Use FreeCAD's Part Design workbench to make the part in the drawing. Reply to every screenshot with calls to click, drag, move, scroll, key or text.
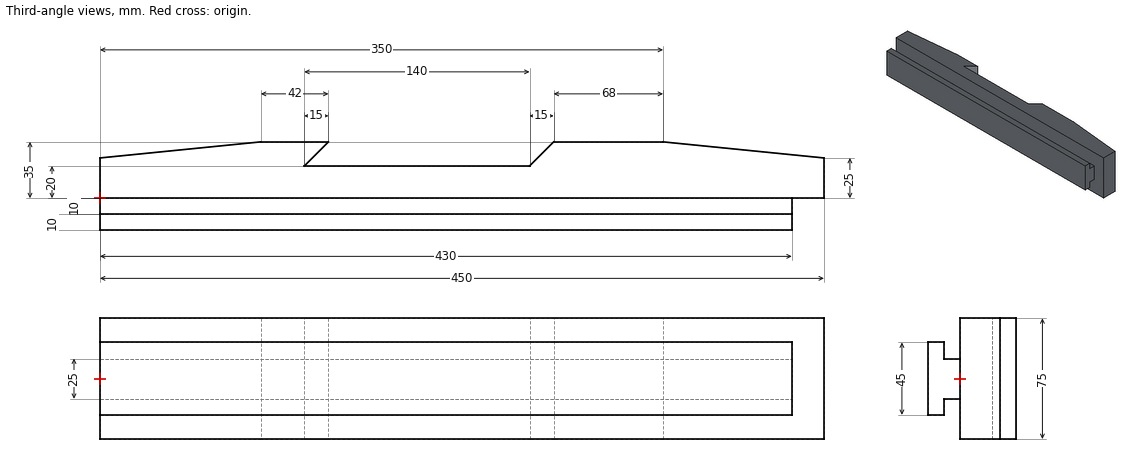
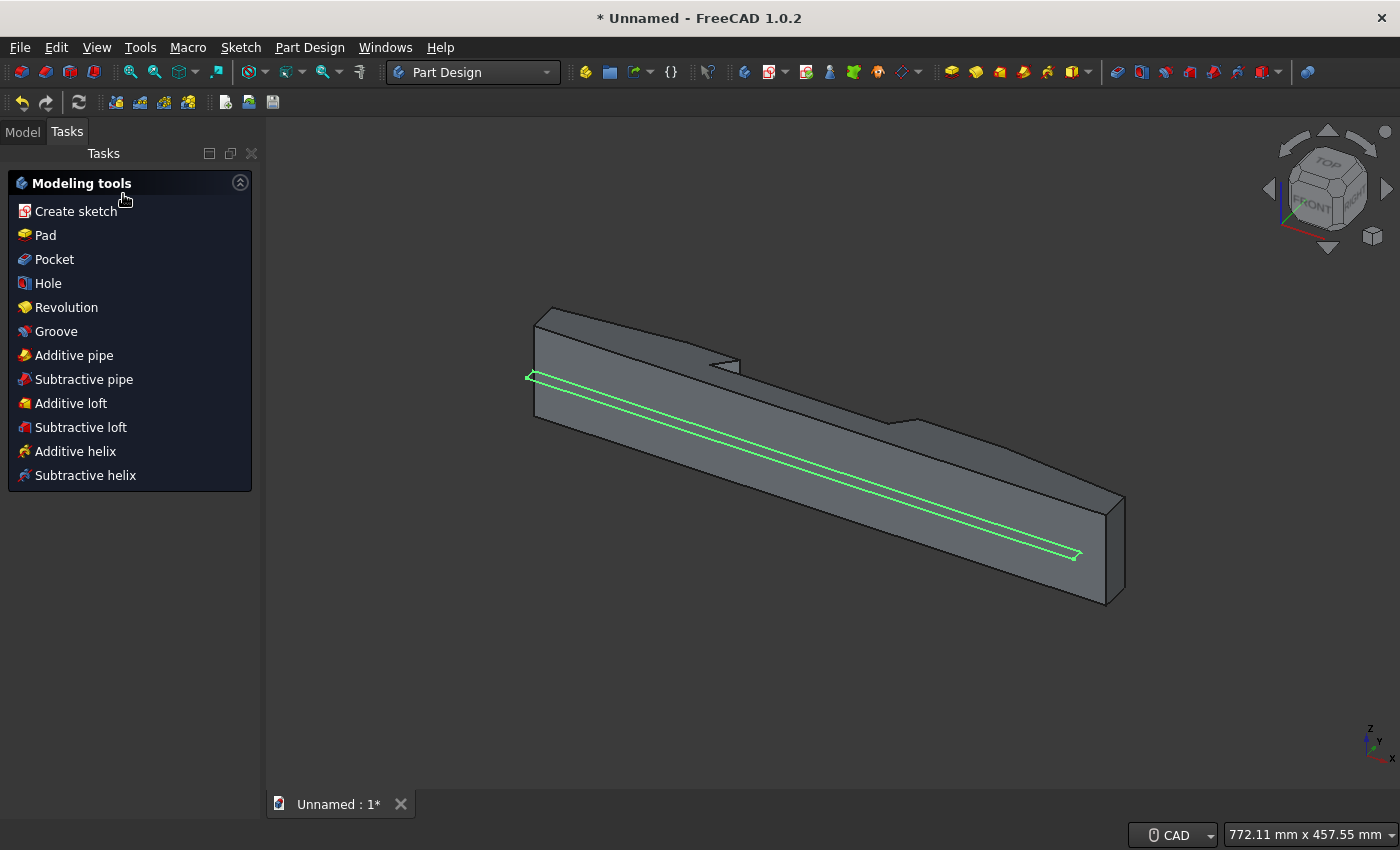
click(952, 72)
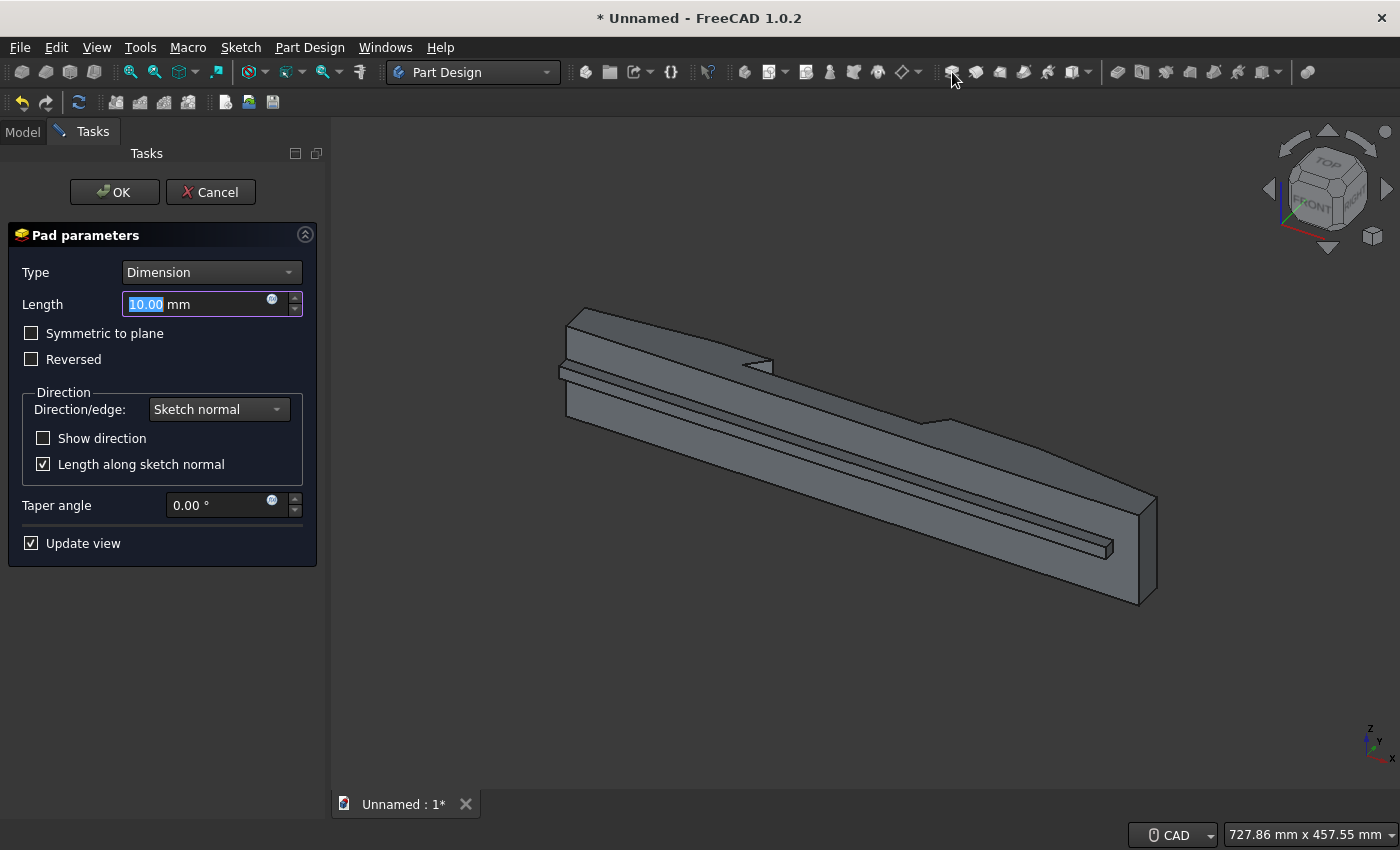
text(25)
key(Tab)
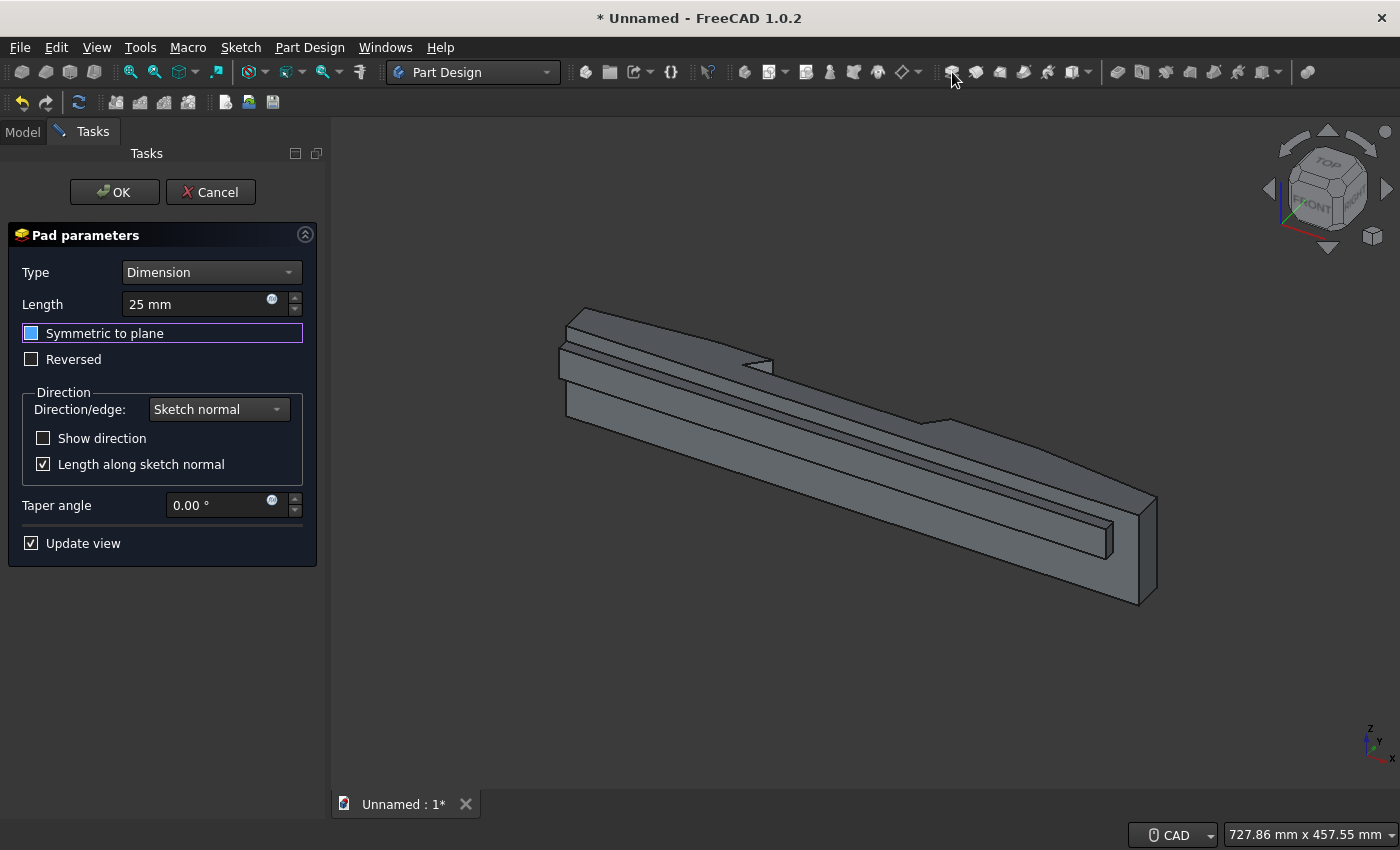
click(30, 333)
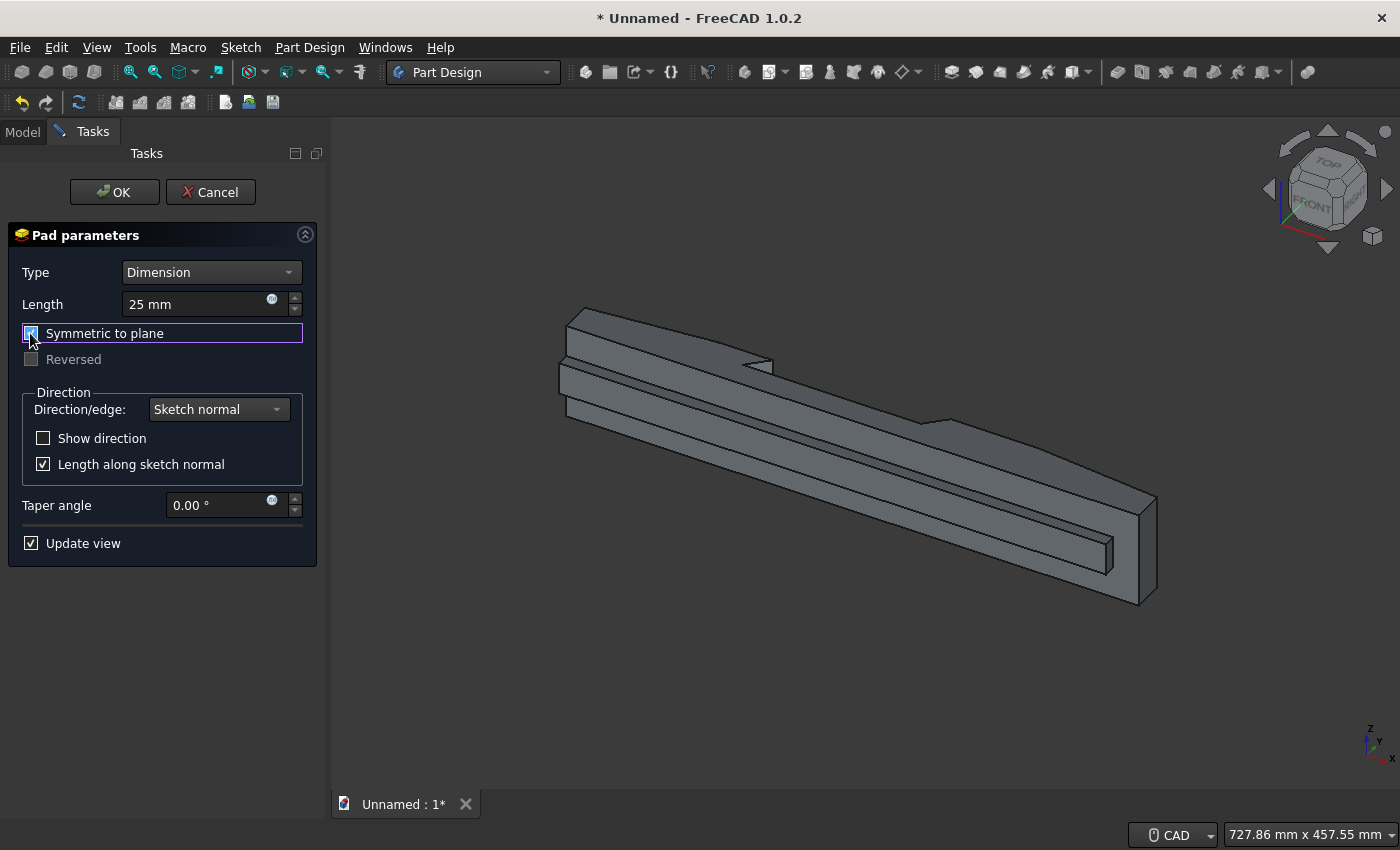
click(115, 192)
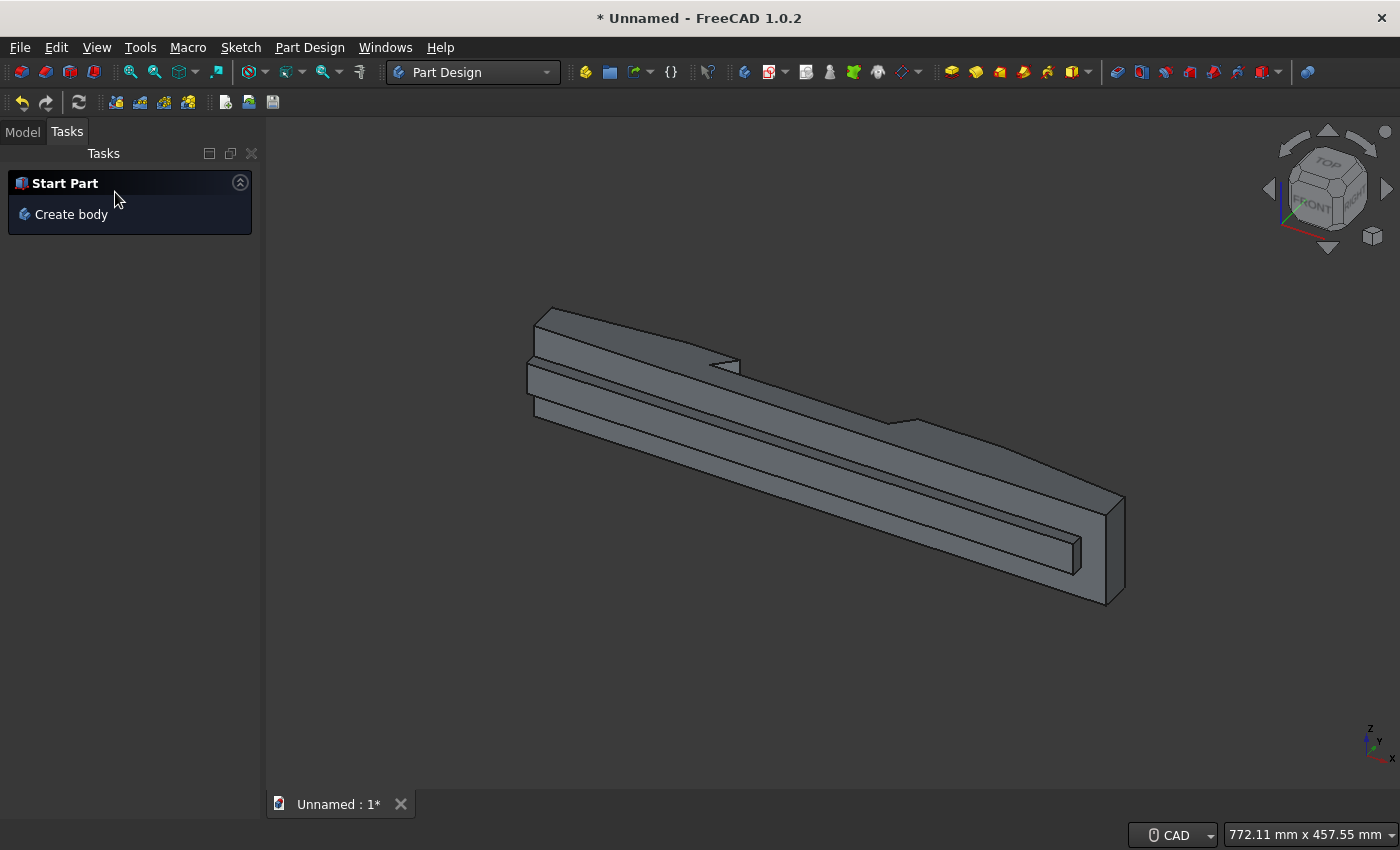
click(770, 72)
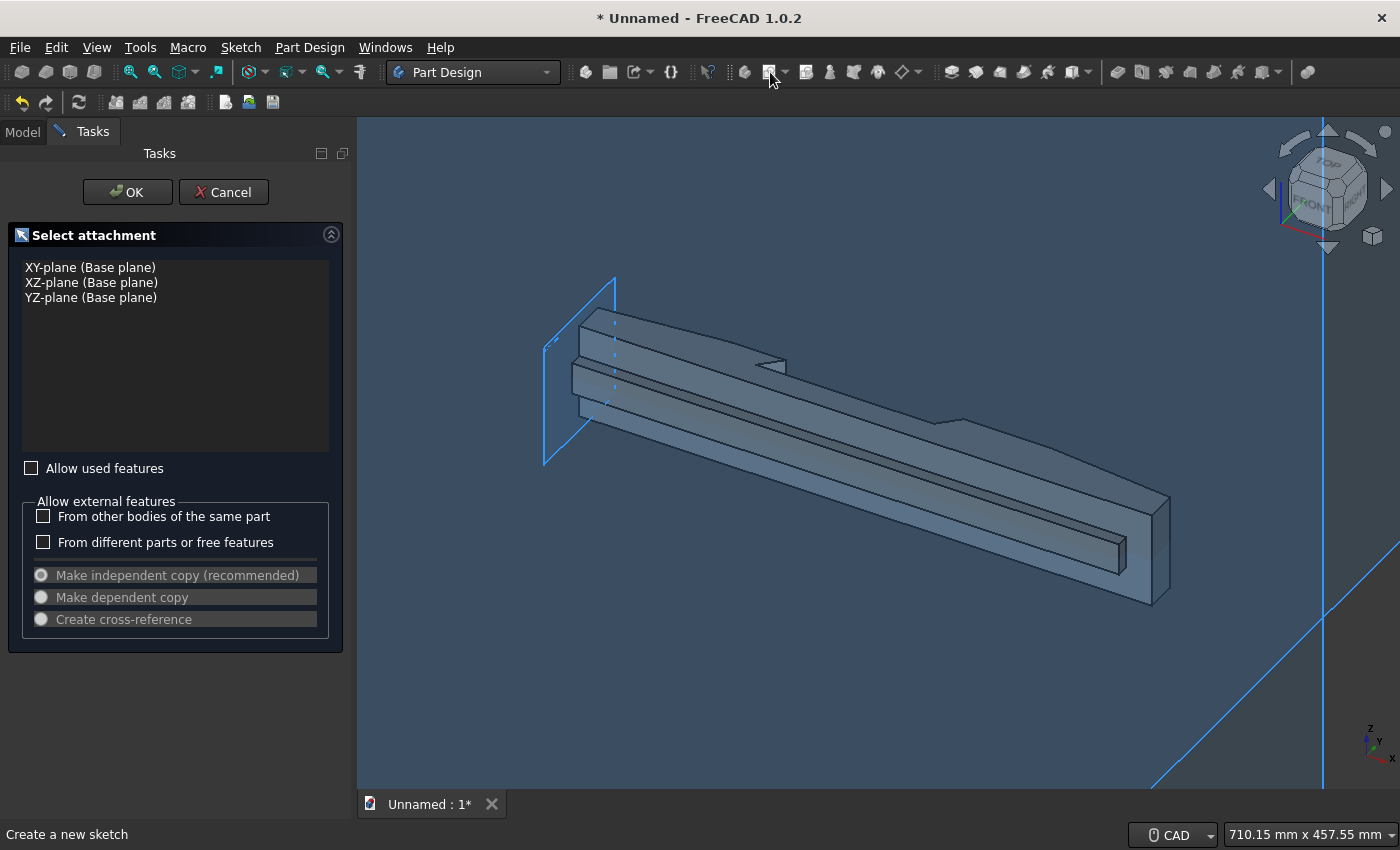
click(82, 268)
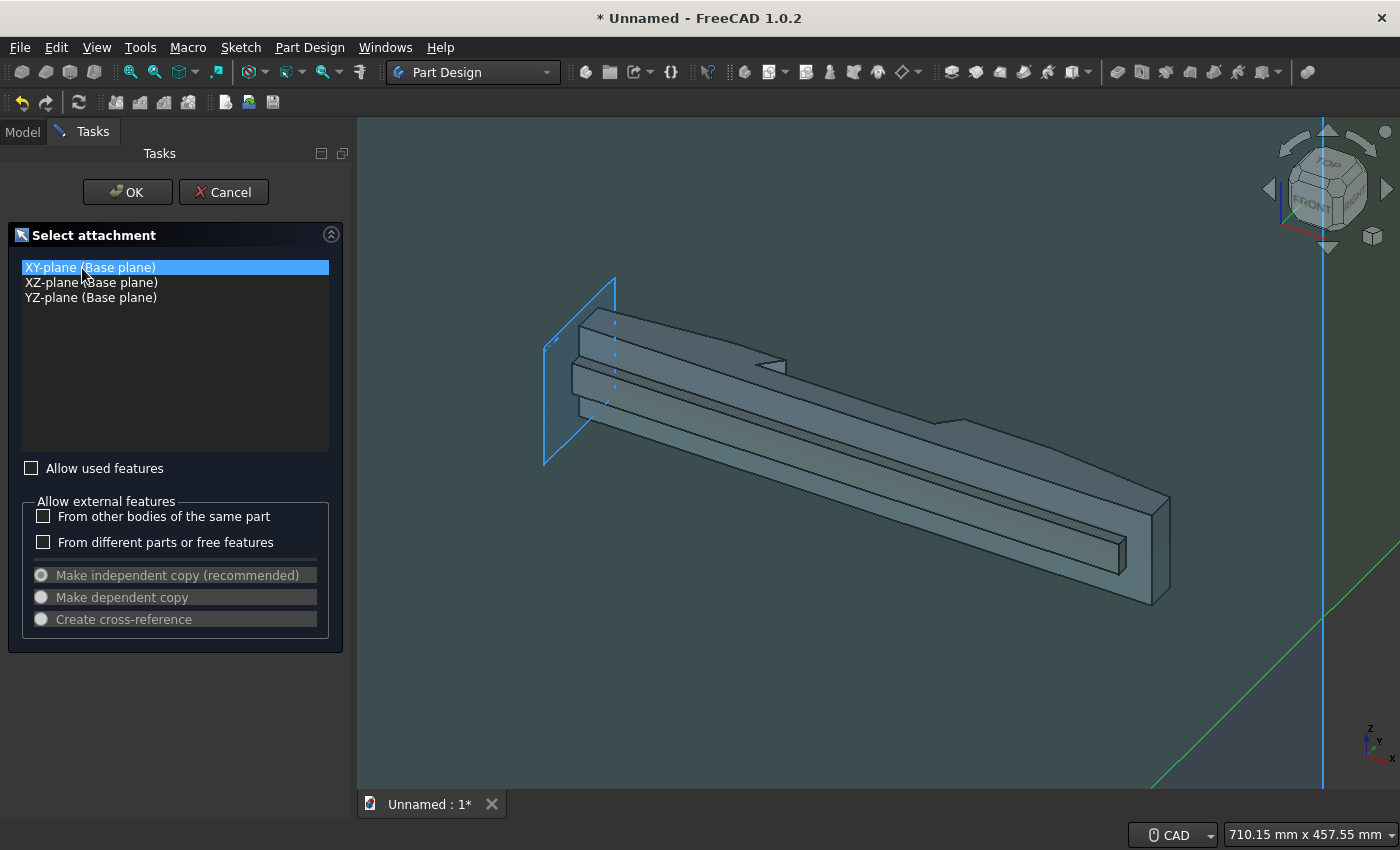
click(128, 192)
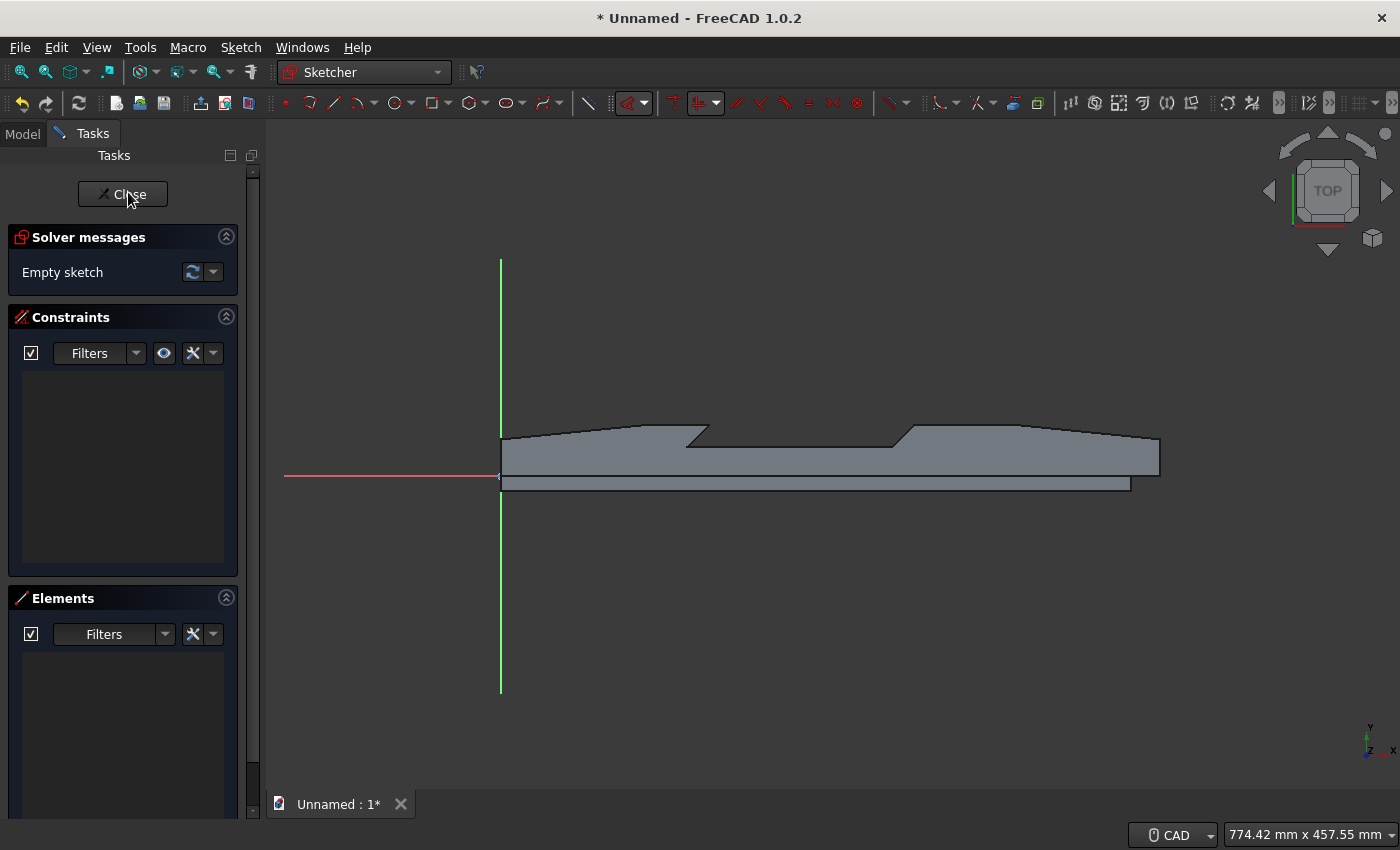
click(250, 104)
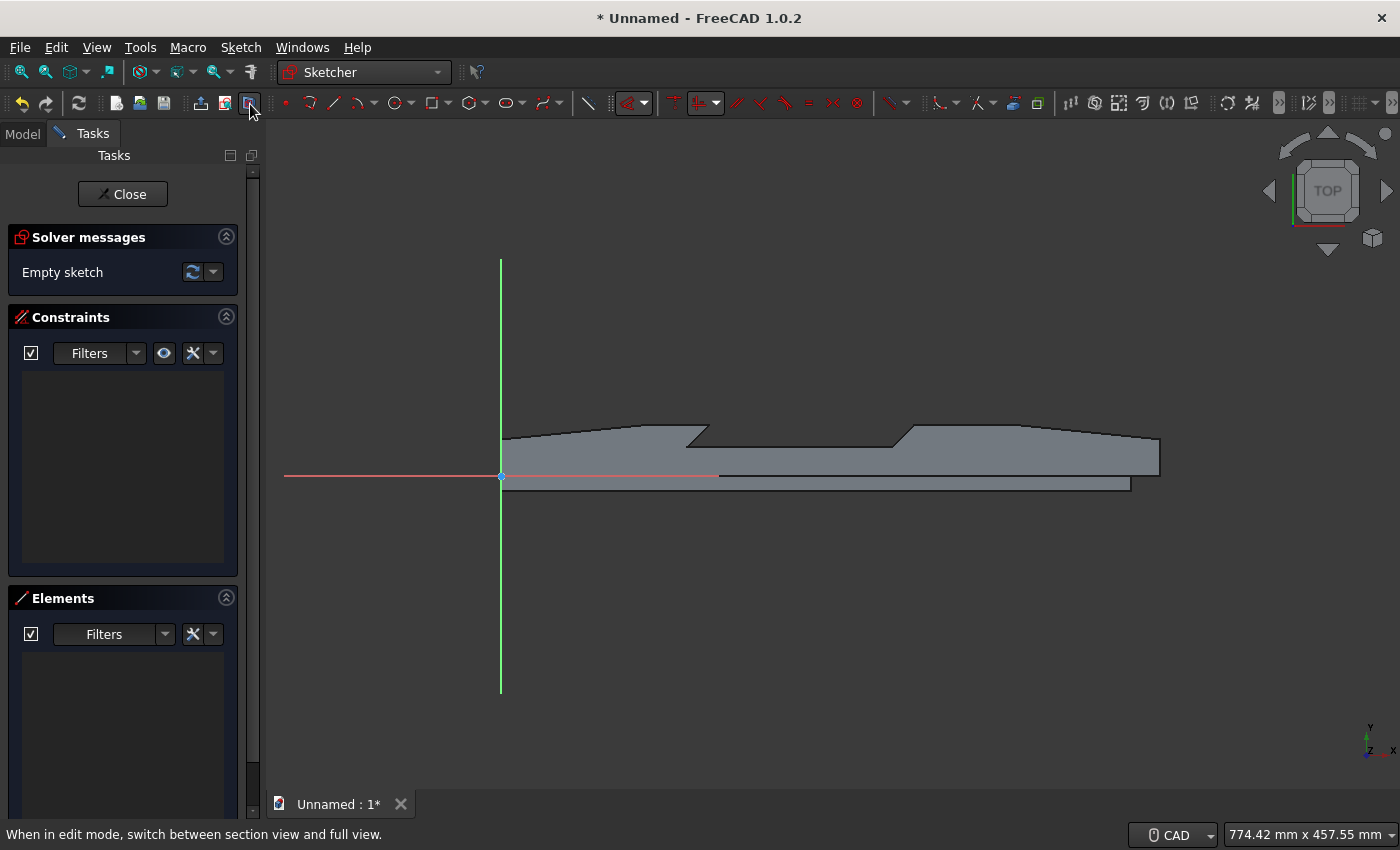
key(g)
key(r)